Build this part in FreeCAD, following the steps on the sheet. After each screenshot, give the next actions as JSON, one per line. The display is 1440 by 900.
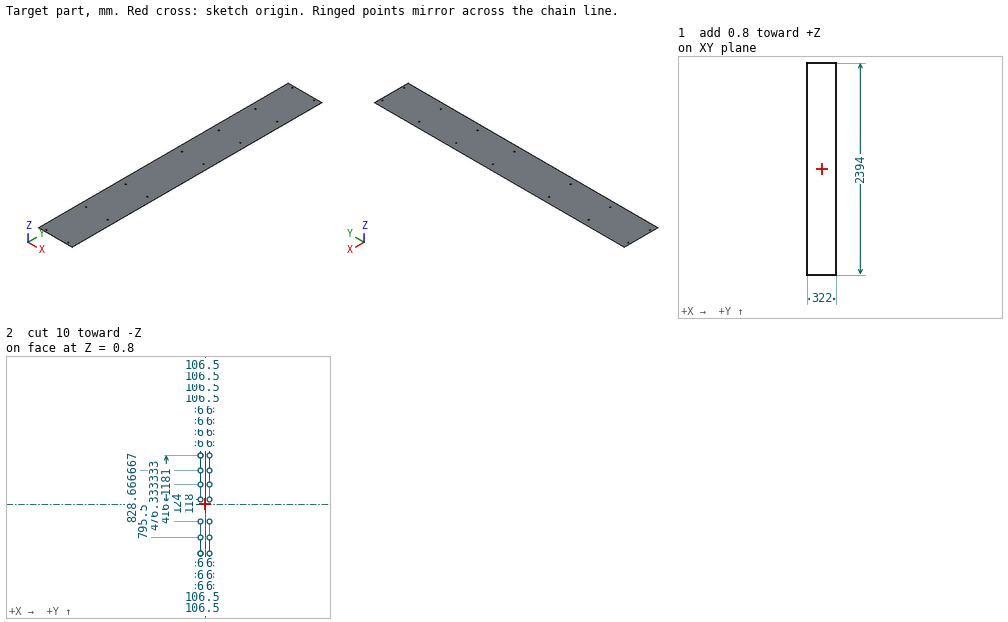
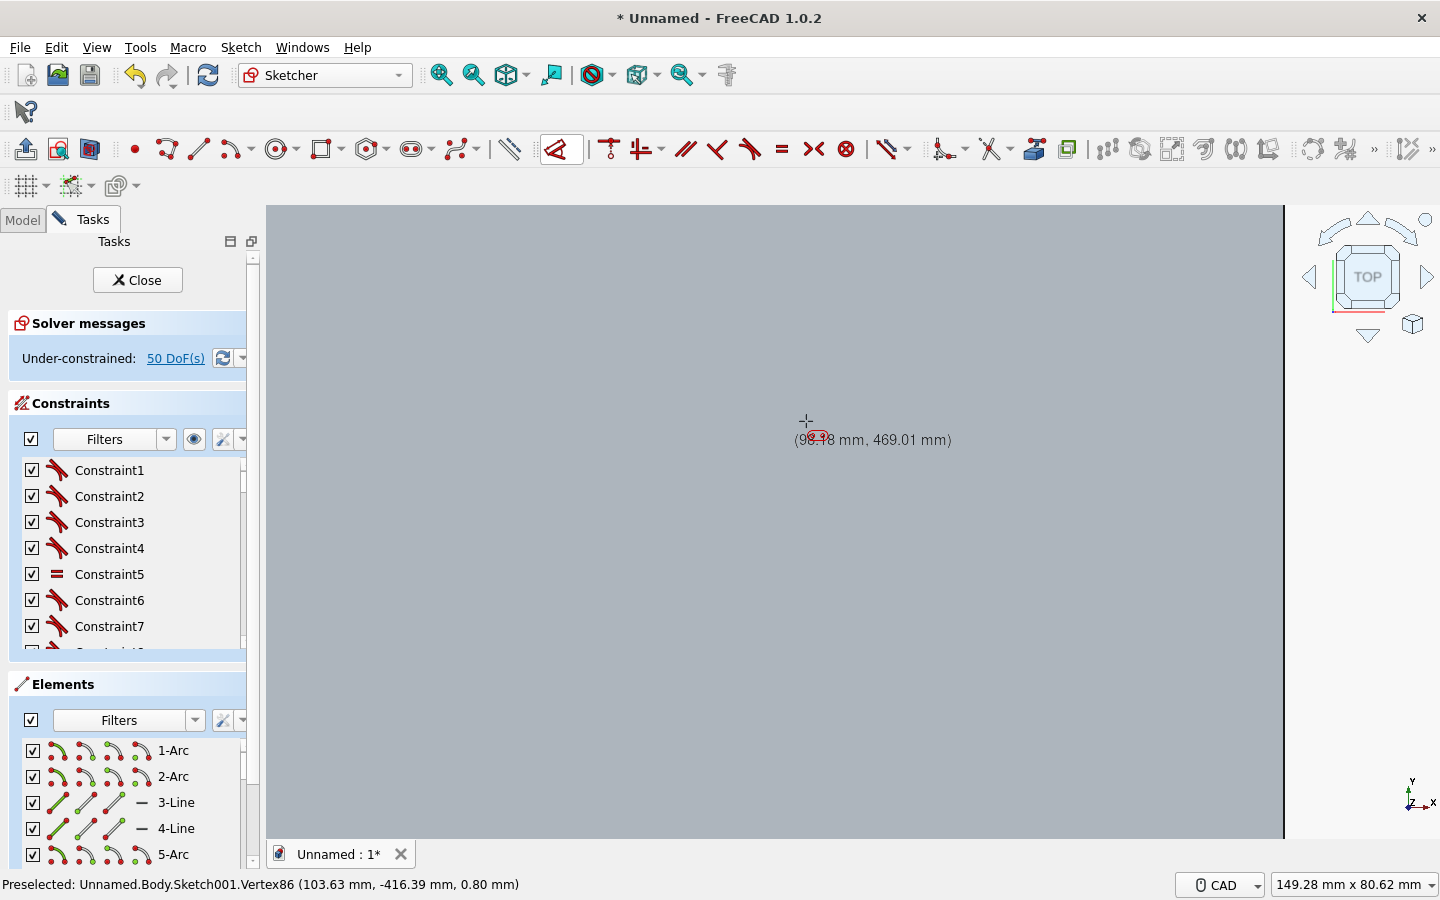
{"action": "scroll", "coordinate": [806, 421], "scroll_direction": "down", "scroll_amount": 18}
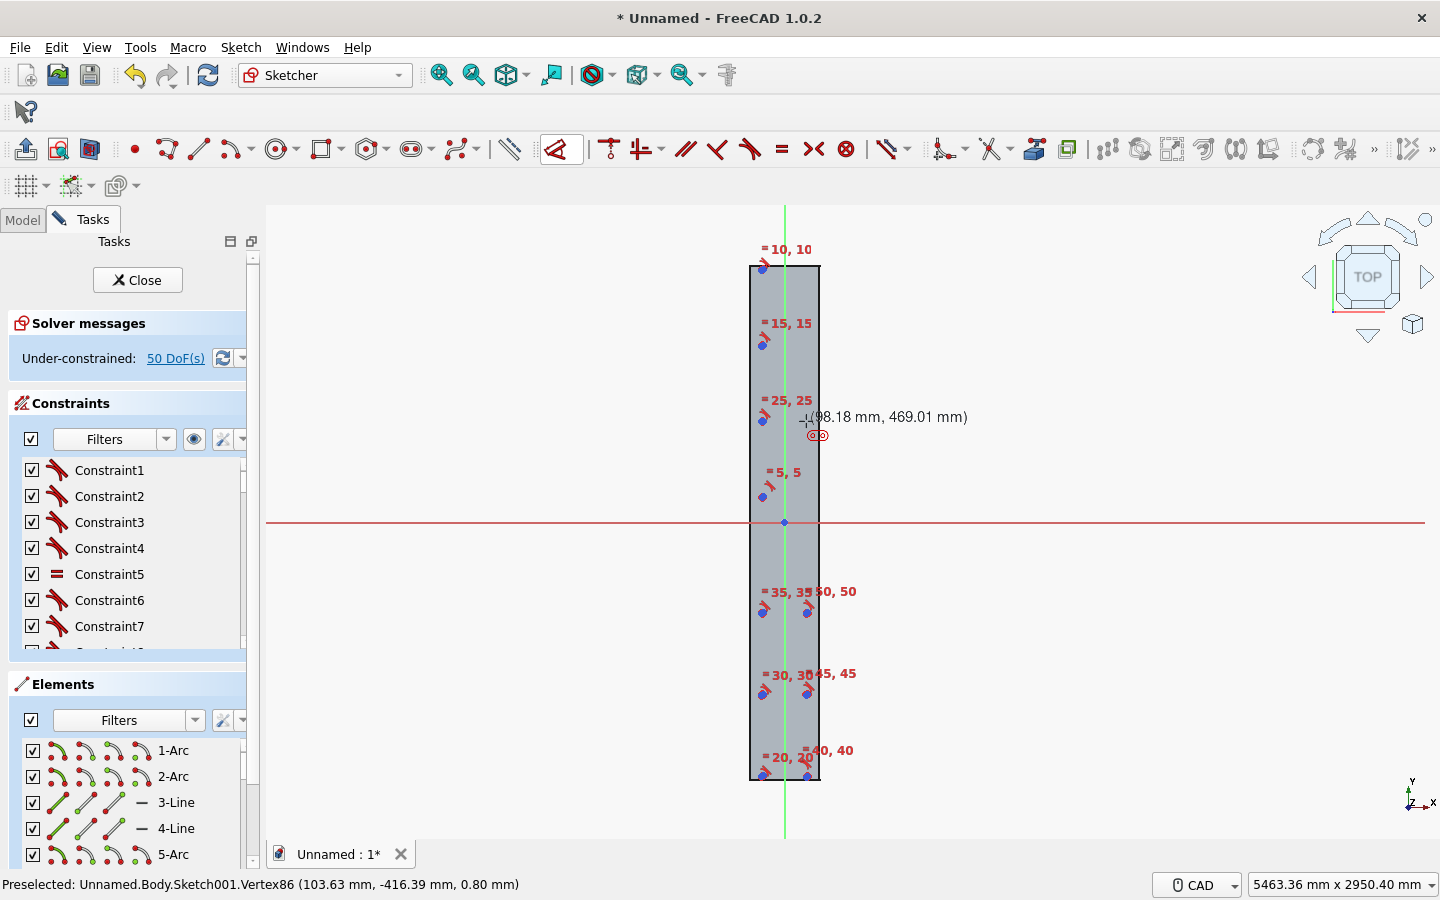
{"action": "left_click", "coordinate": [806, 421]}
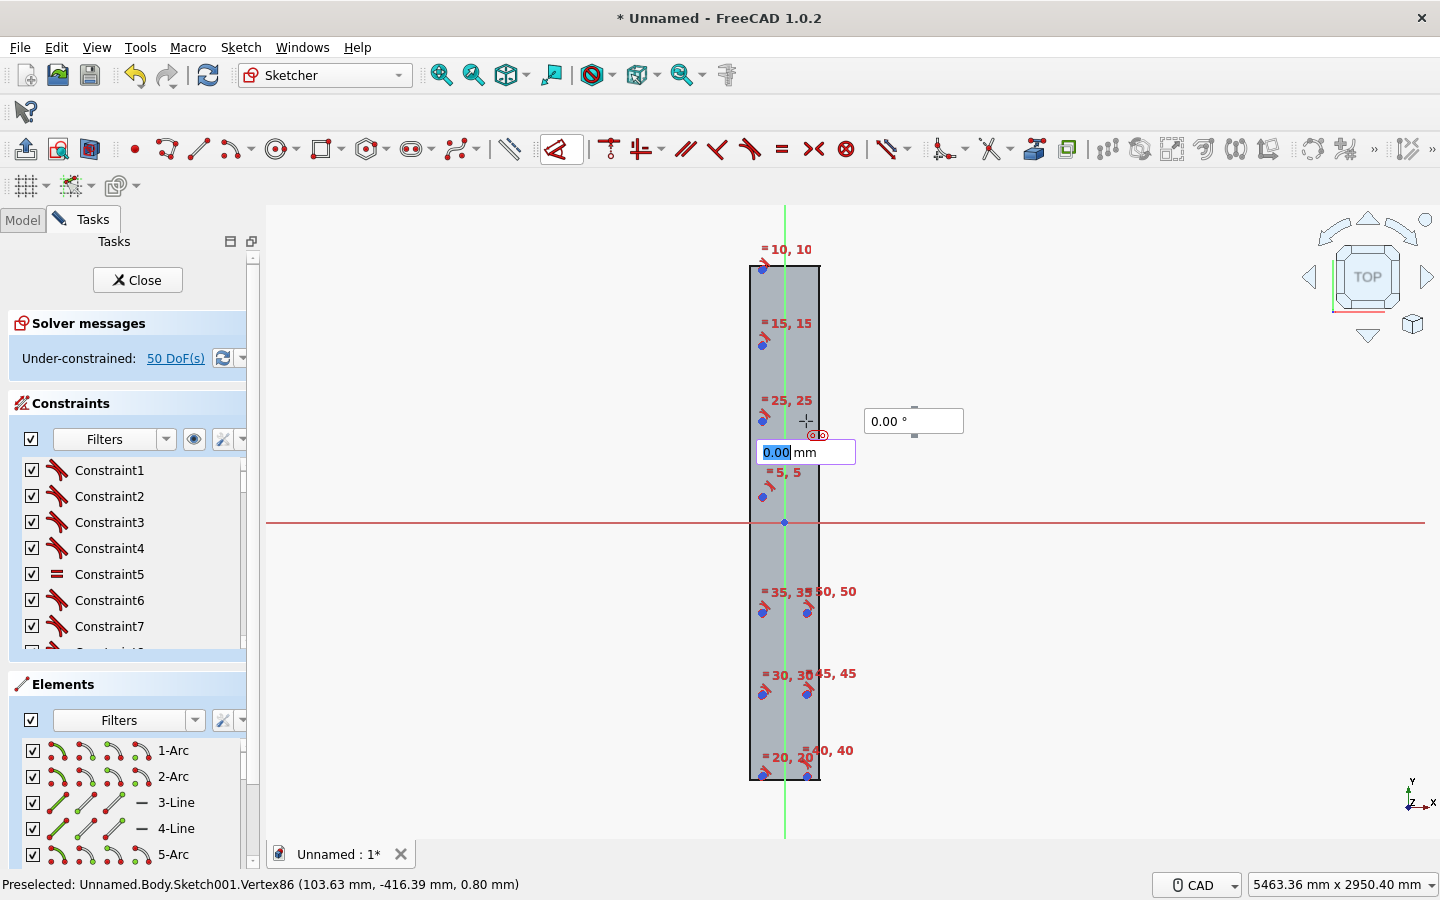
{"action": "scroll", "coordinate": [808, 421], "scroll_direction": "up", "scroll_amount": 13}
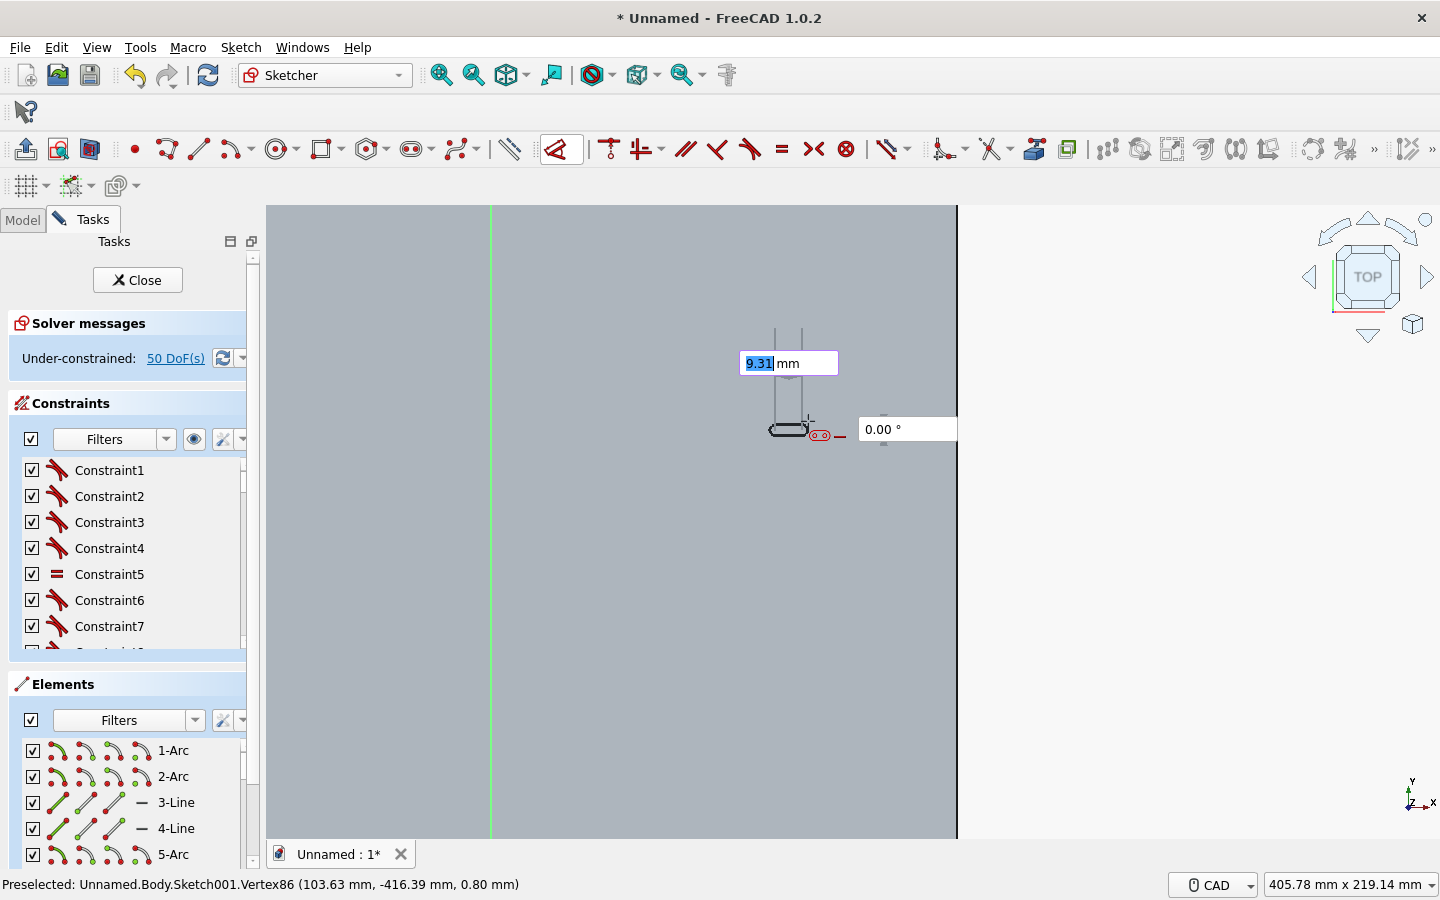
{"action": "left_click", "coordinate": [799, 417]}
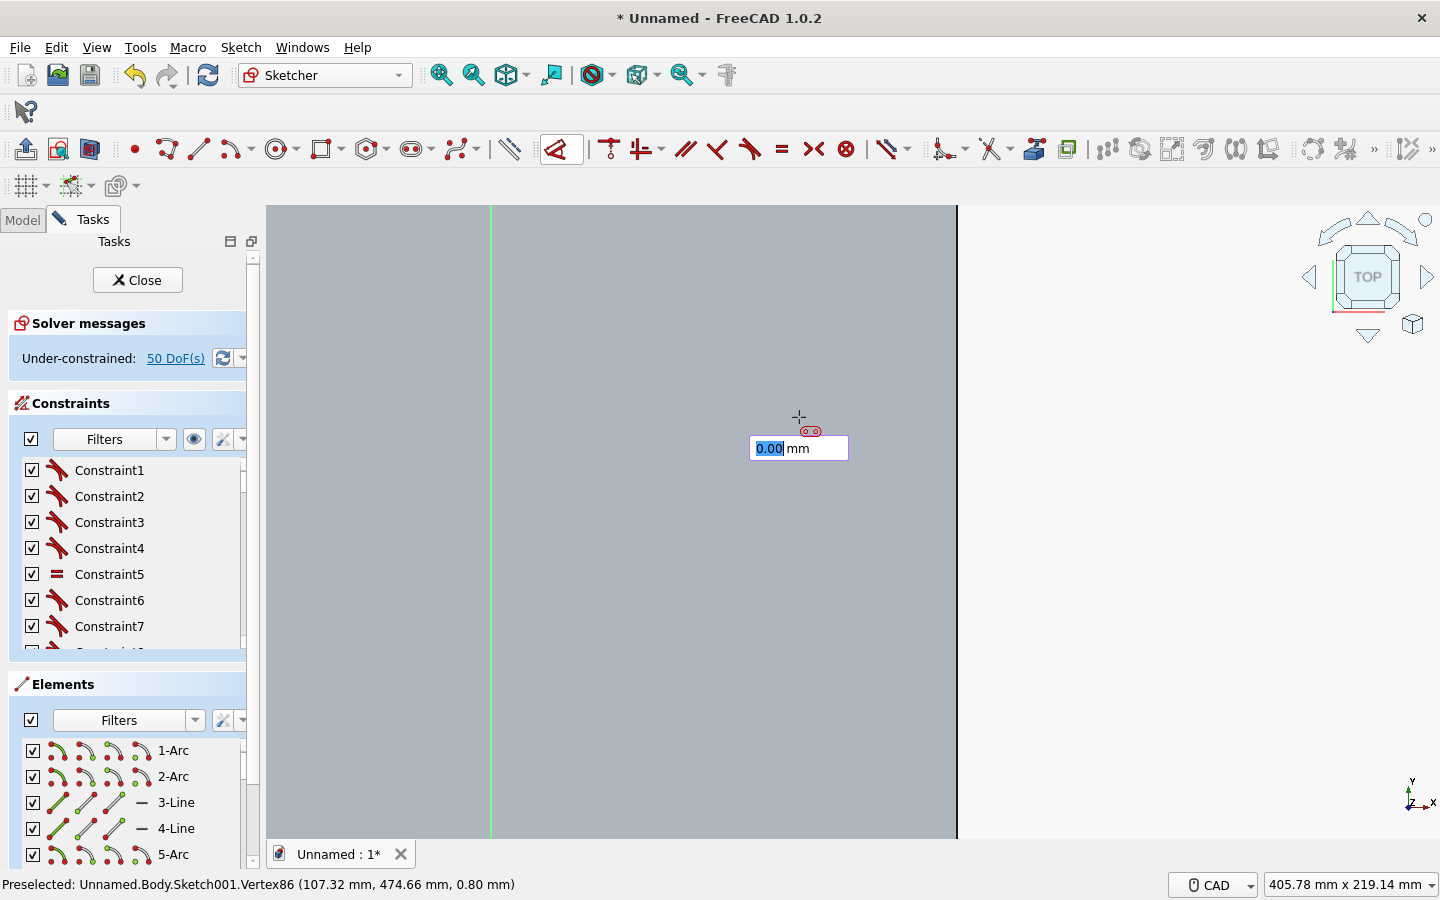
{"action": "scroll", "coordinate": [791, 409], "scroll_direction": "up", "scroll_amount": 4}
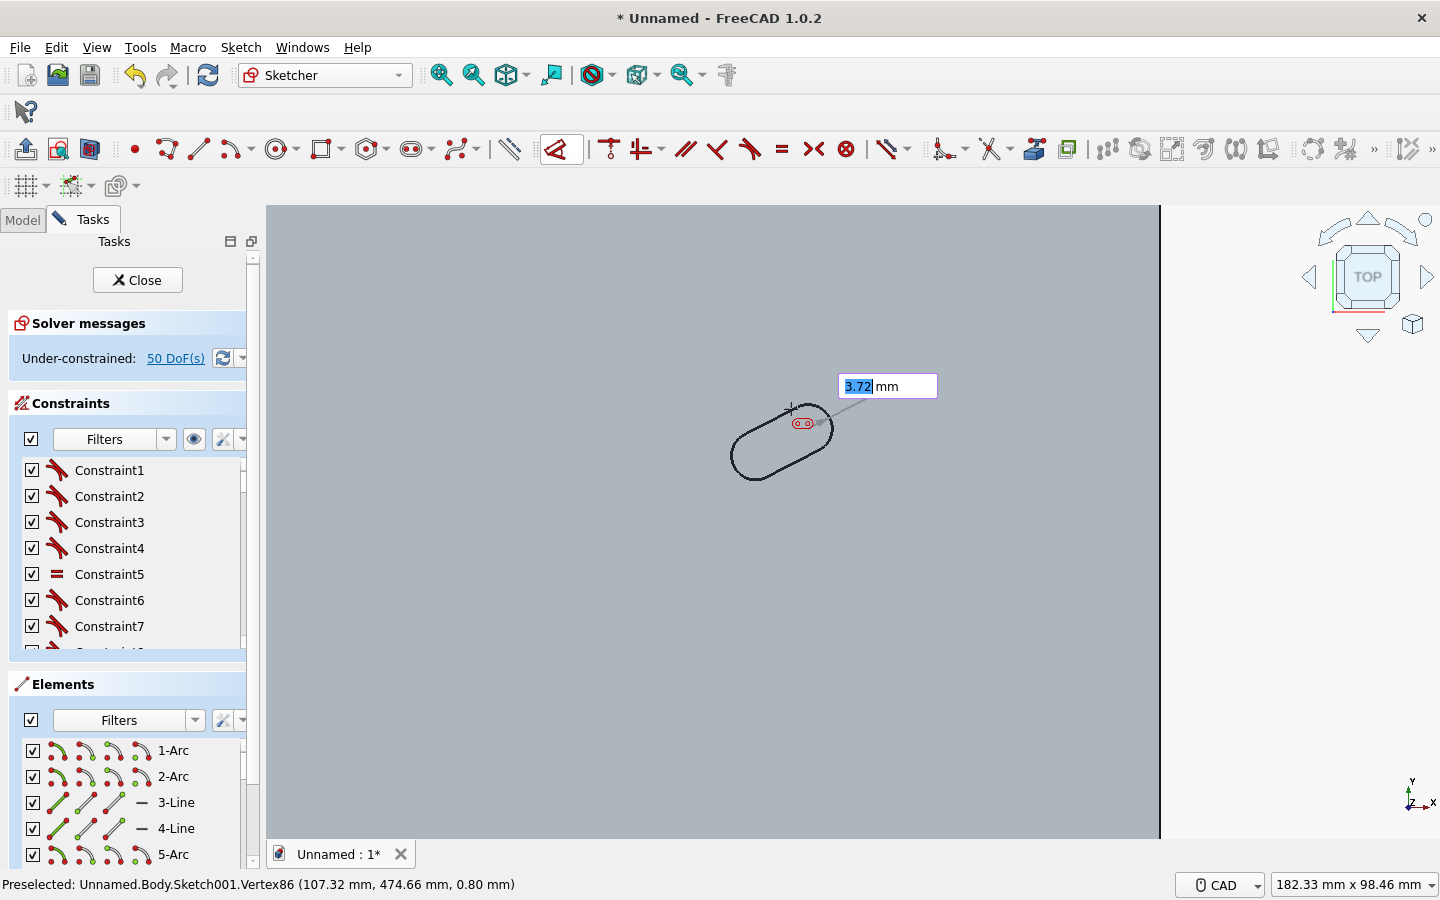
{"action": "left_click", "coordinate": [790, 409]}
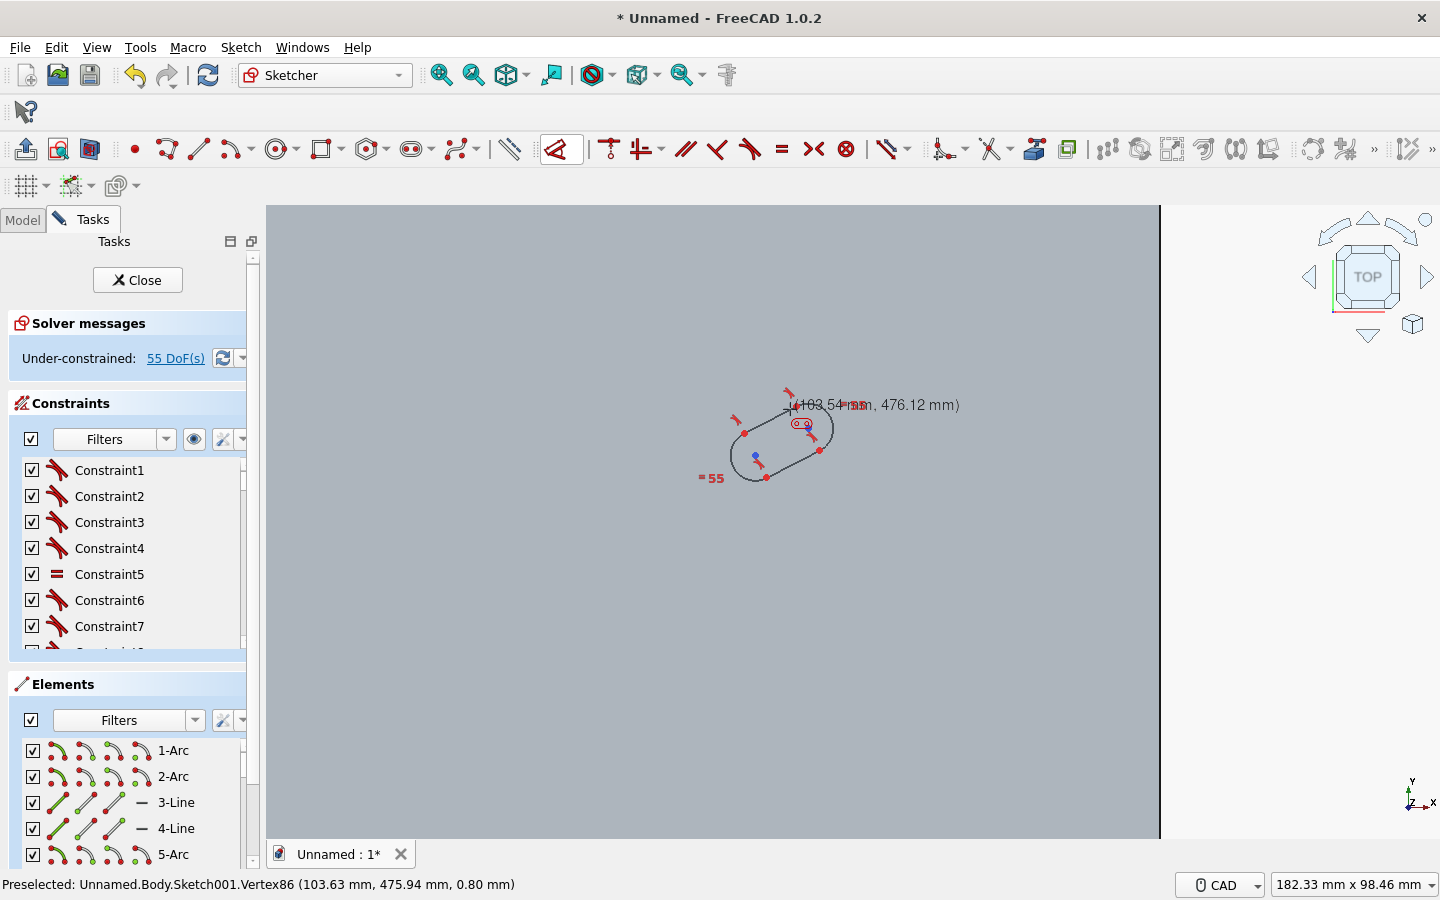
{"action": "scroll", "coordinate": [807, 420], "scroll_direction": "down", "scroll_amount": 17}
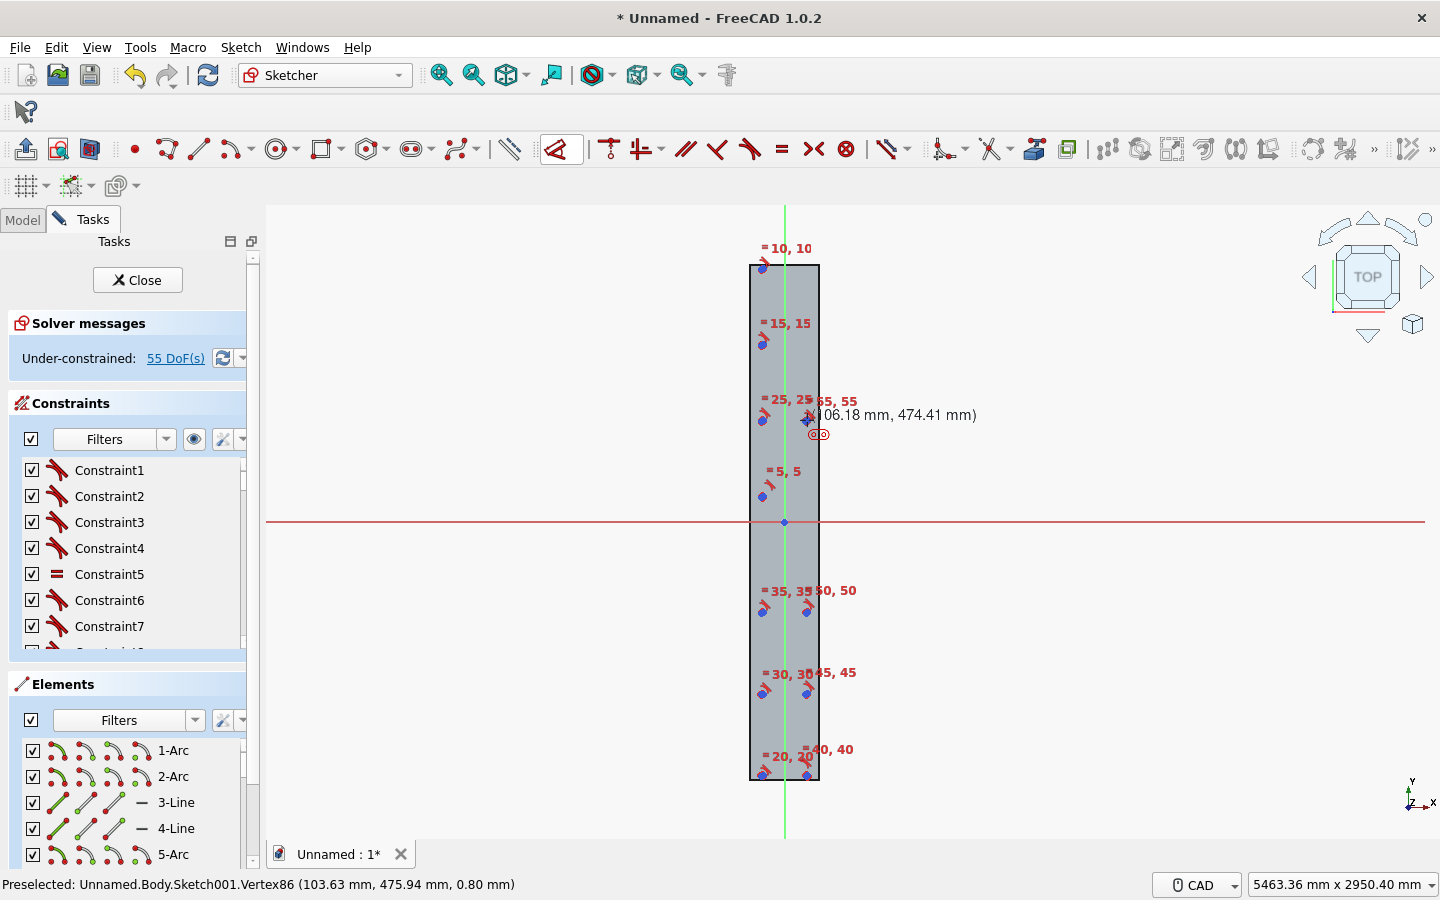
{"action": "scroll", "coordinate": [806, 345], "scroll_direction": "up", "scroll_amount": 18}